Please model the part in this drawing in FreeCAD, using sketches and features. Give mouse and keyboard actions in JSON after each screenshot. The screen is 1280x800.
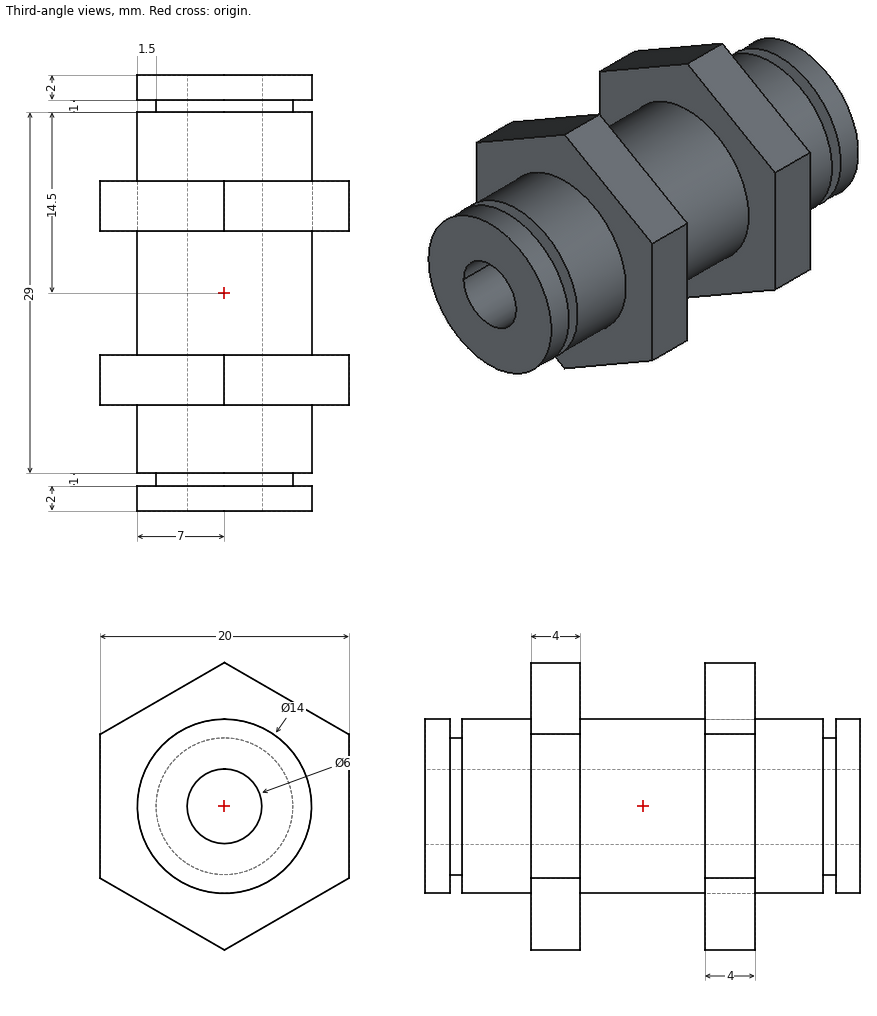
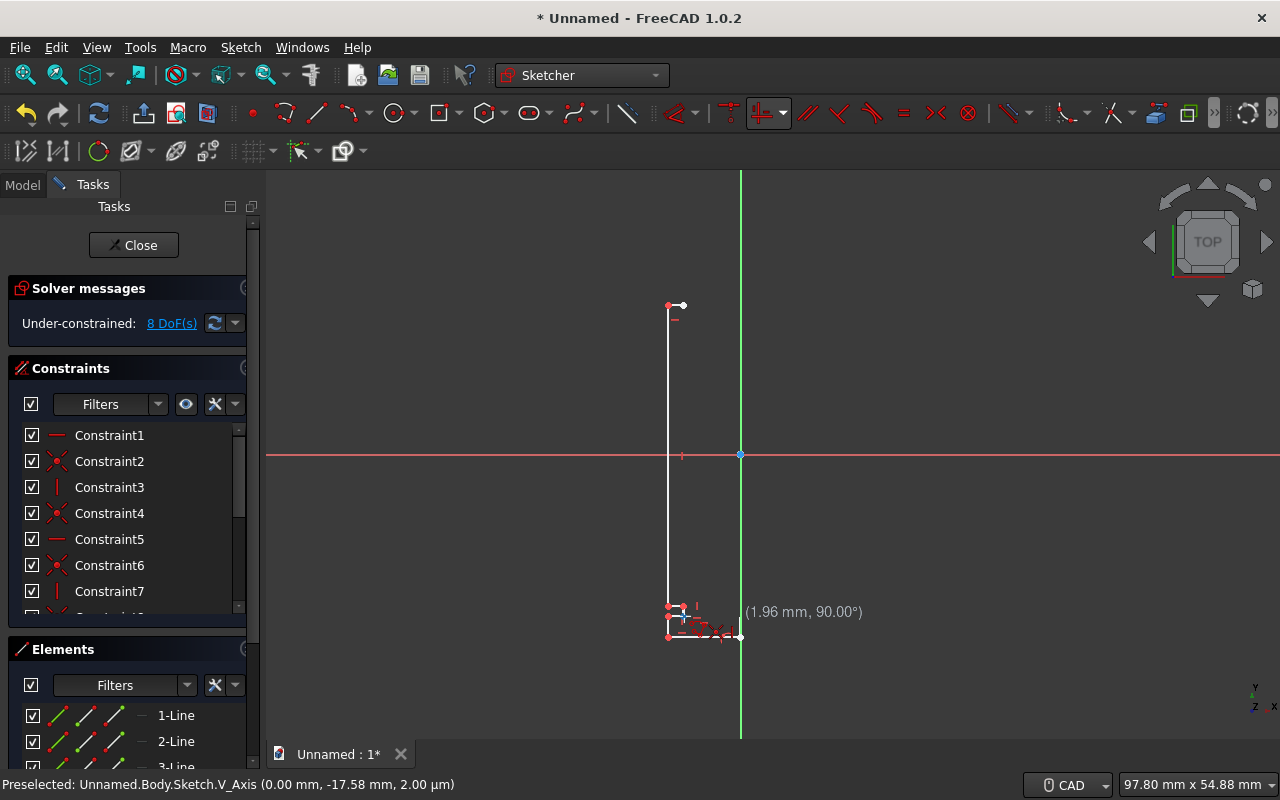
{"action": "left_click", "coordinate": [732, 274]}
{"action": "left_click", "coordinate": [668, 274]}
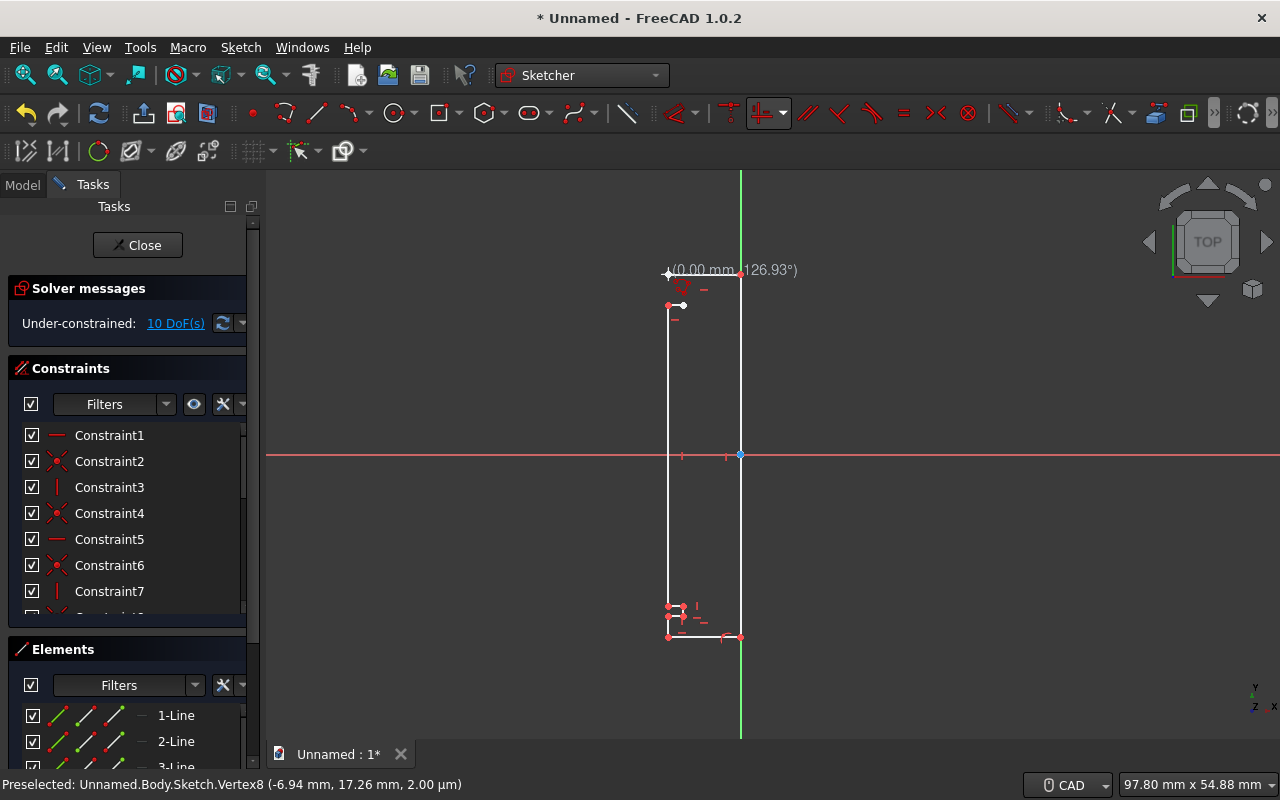
{"action": "scroll", "coordinate": [668, 294], "scroll_direction": "up", "scroll_amount": 3}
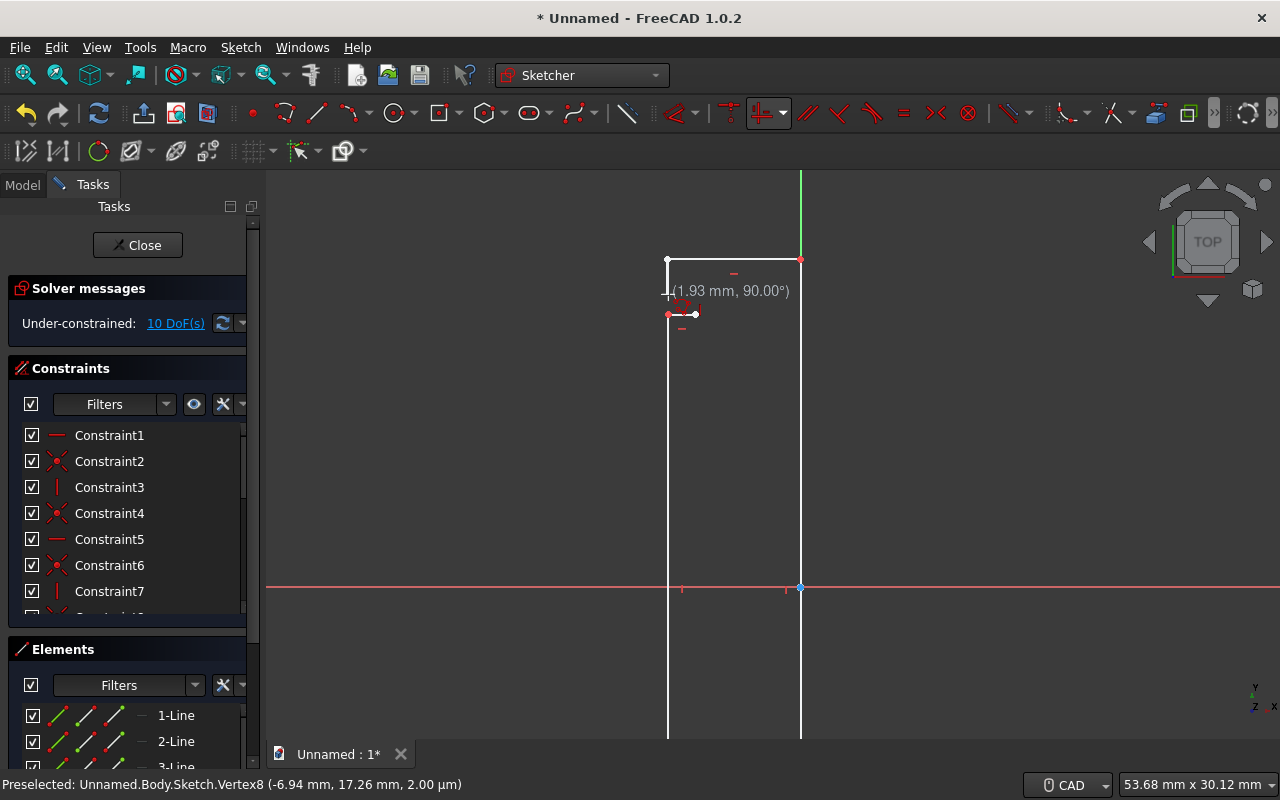
{"action": "left_click", "coordinate": [668, 294]}
{"action": "left_click", "coordinate": [697, 294]}
{"action": "left_click", "coordinate": [696, 315]}
{"action": "key", "text": "Escape"}
{"action": "key", "text": "Escape"}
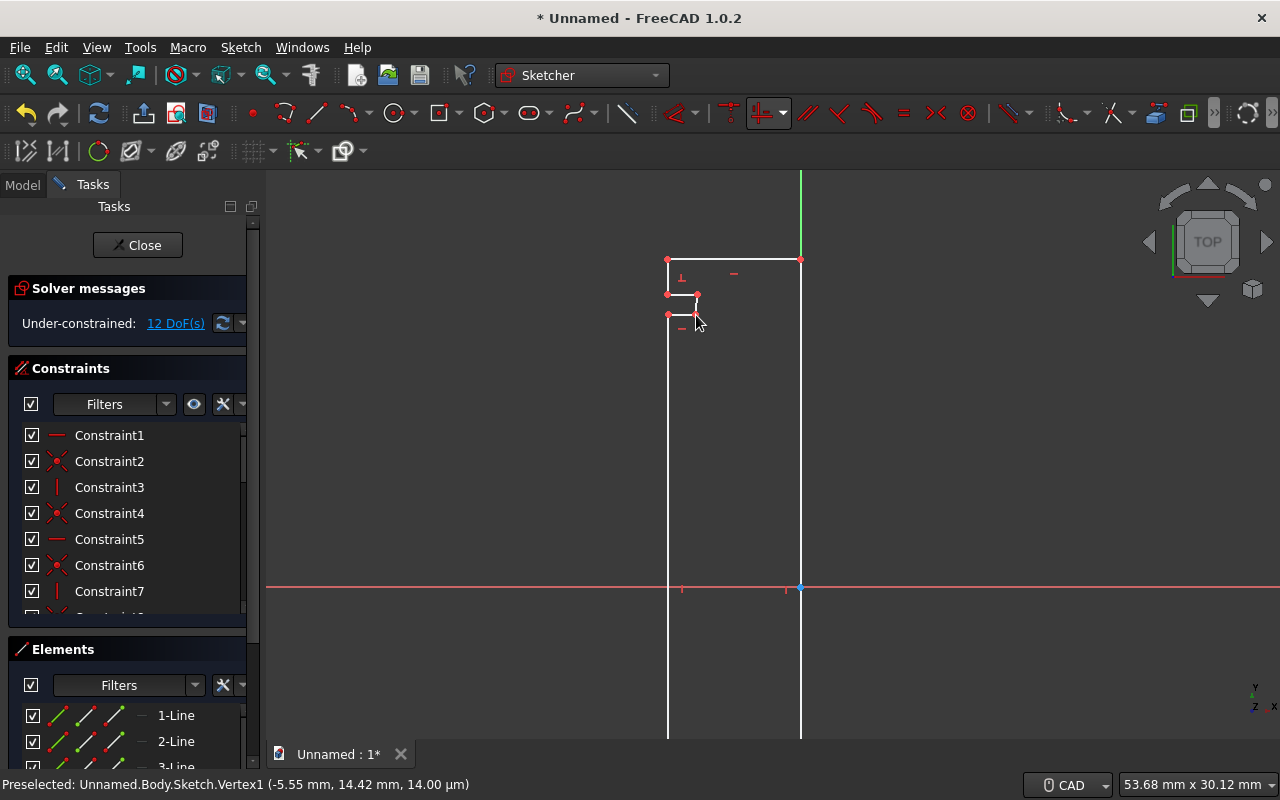
{"action": "scroll", "coordinate": [696, 305], "scroll_direction": "up", "scroll_amount": 2}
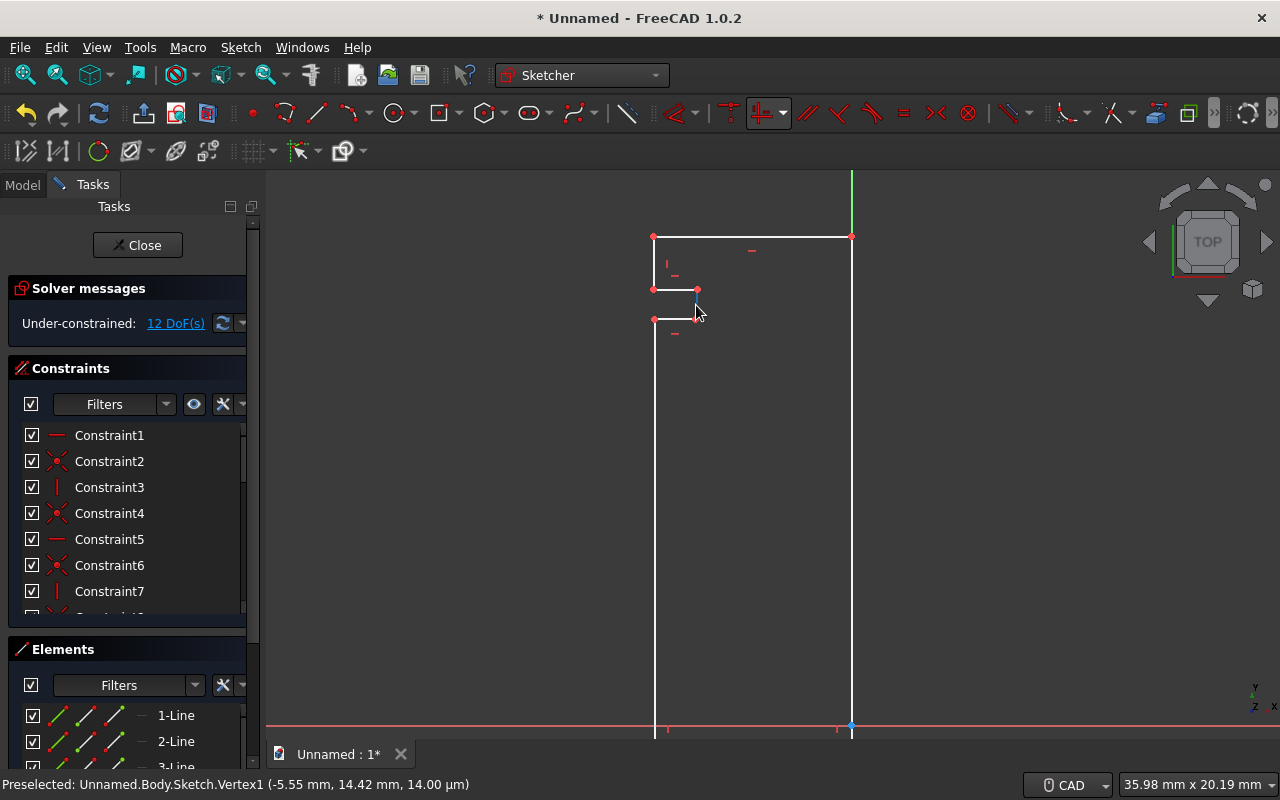
{"action": "left_click", "coordinate": [696, 305]}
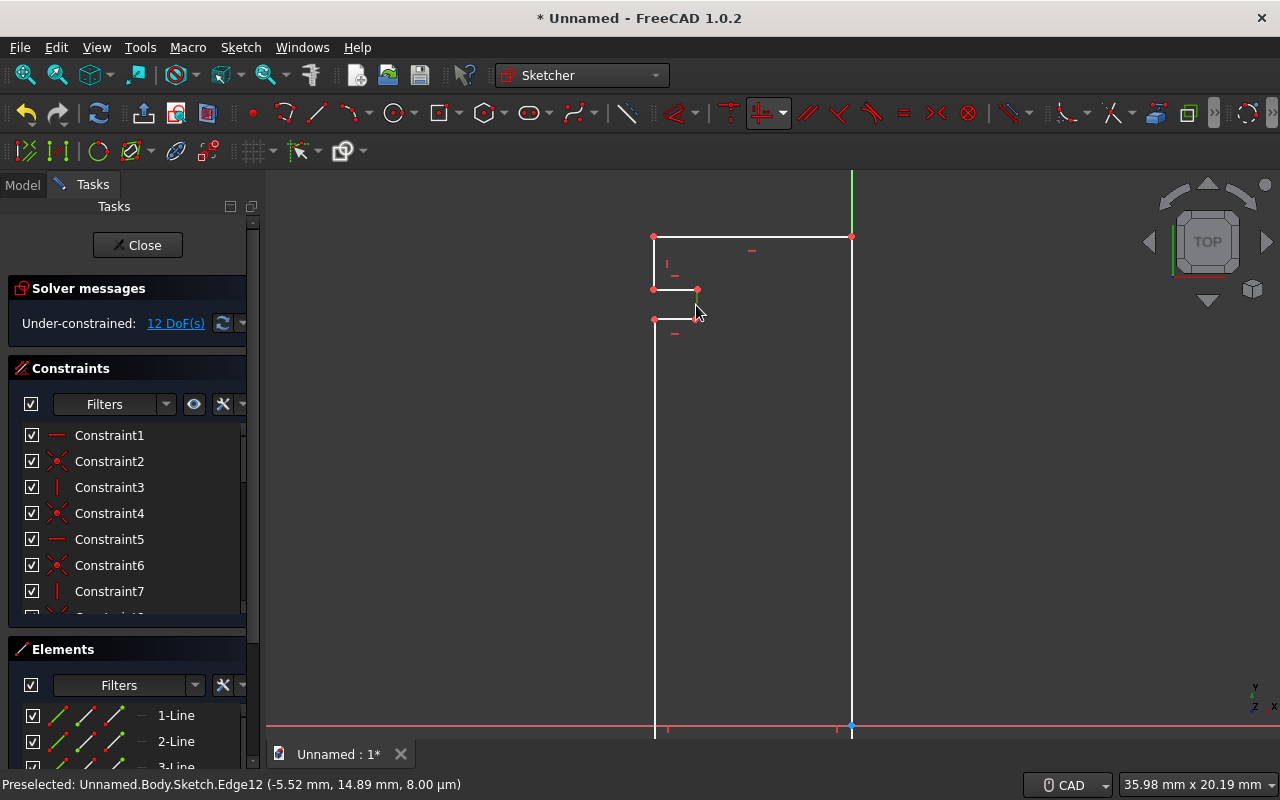
{"action": "key", "text": "v"}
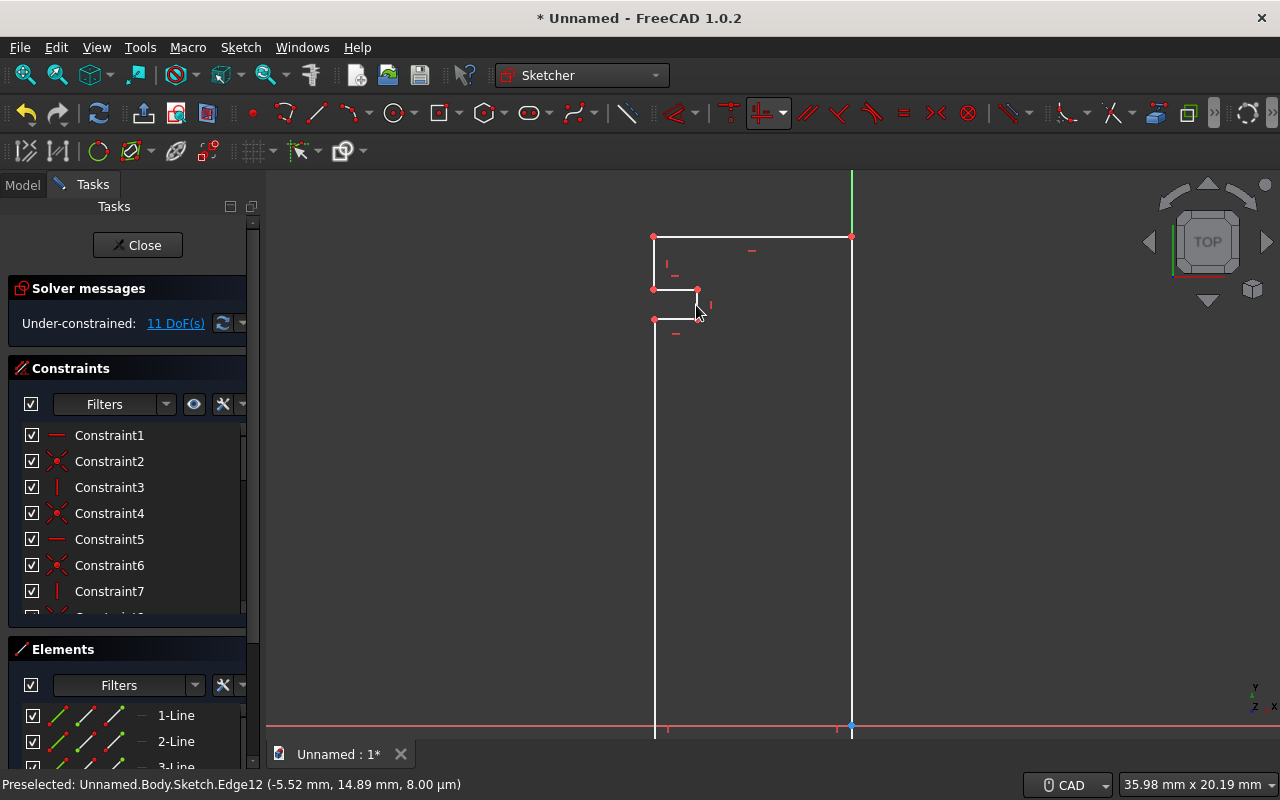
{"action": "scroll", "coordinate": [676, 297], "scroll_direction": "down", "scroll_amount": 5}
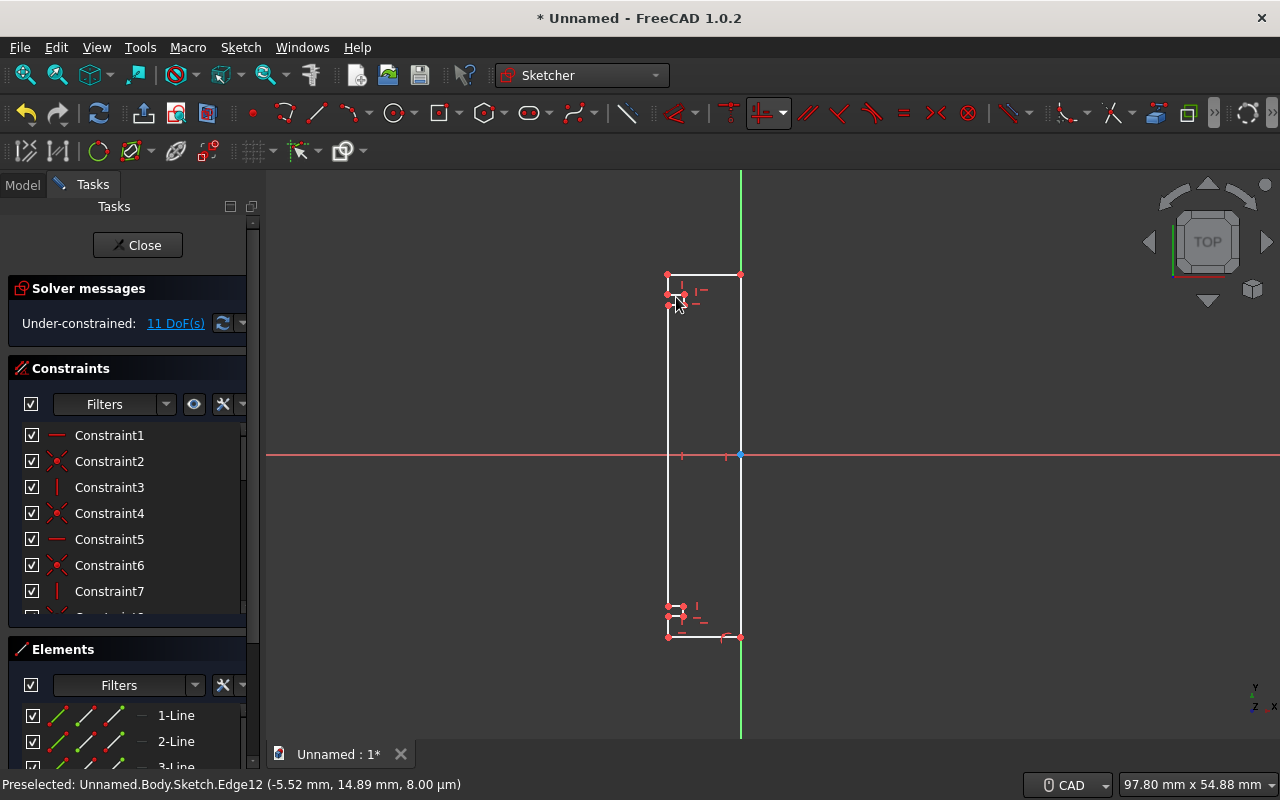
{"action": "scroll", "coordinate": [683, 610], "scroll_direction": "up", "scroll_amount": 7}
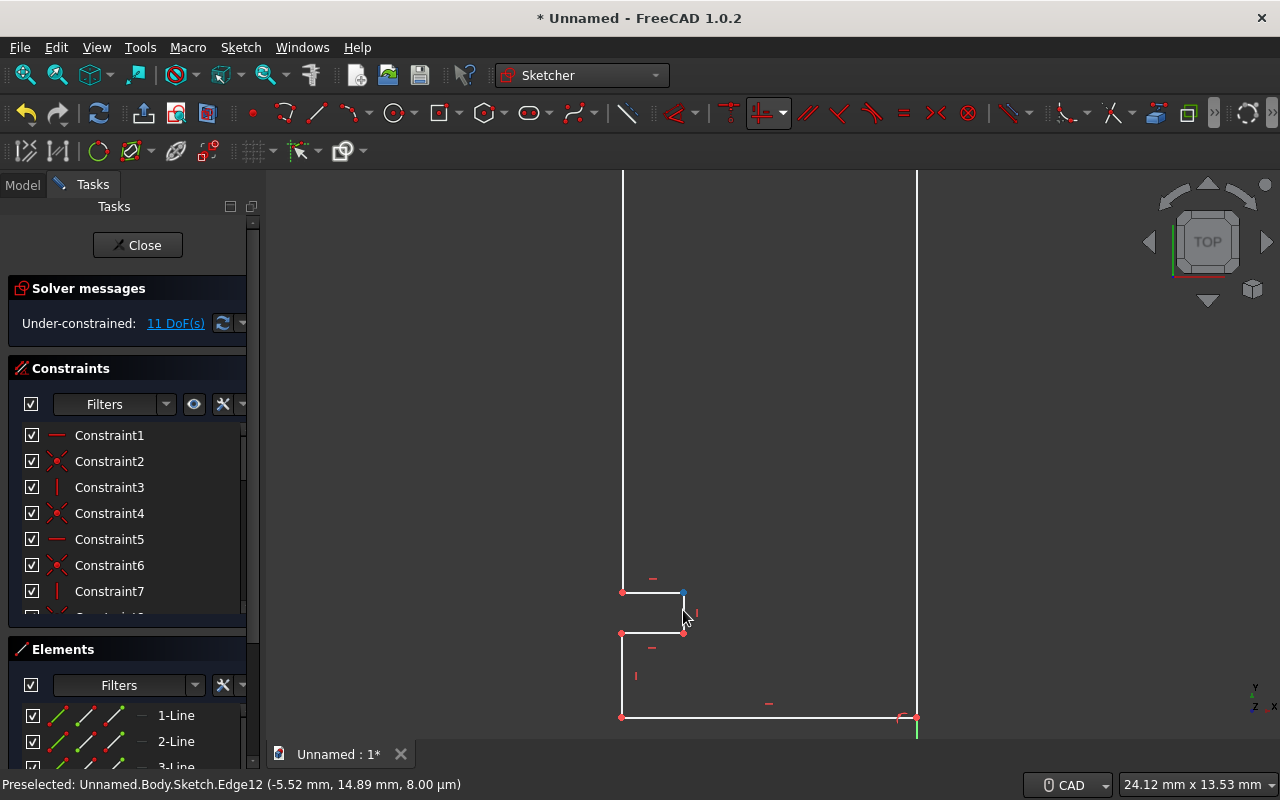
{"action": "left_click", "coordinate": [684, 609]}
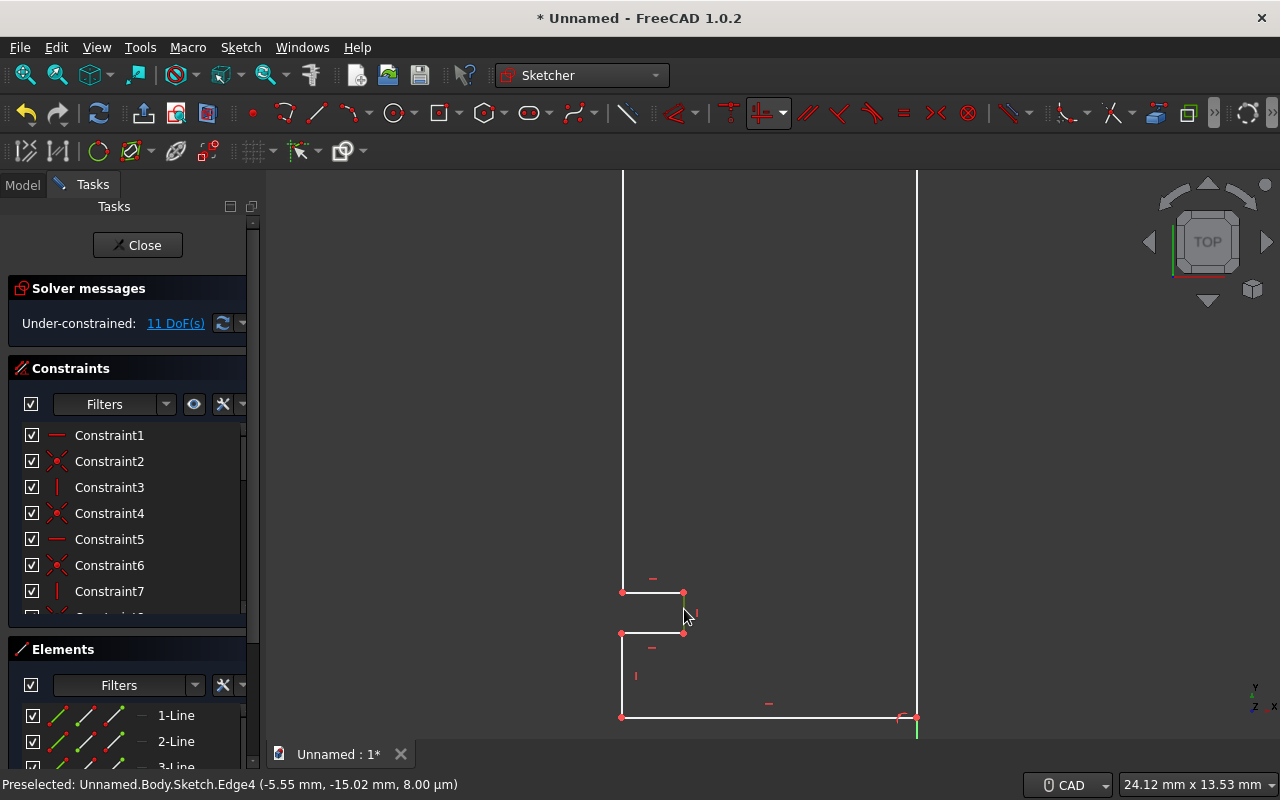
{"action": "left_click", "coordinate": [698, 114]}